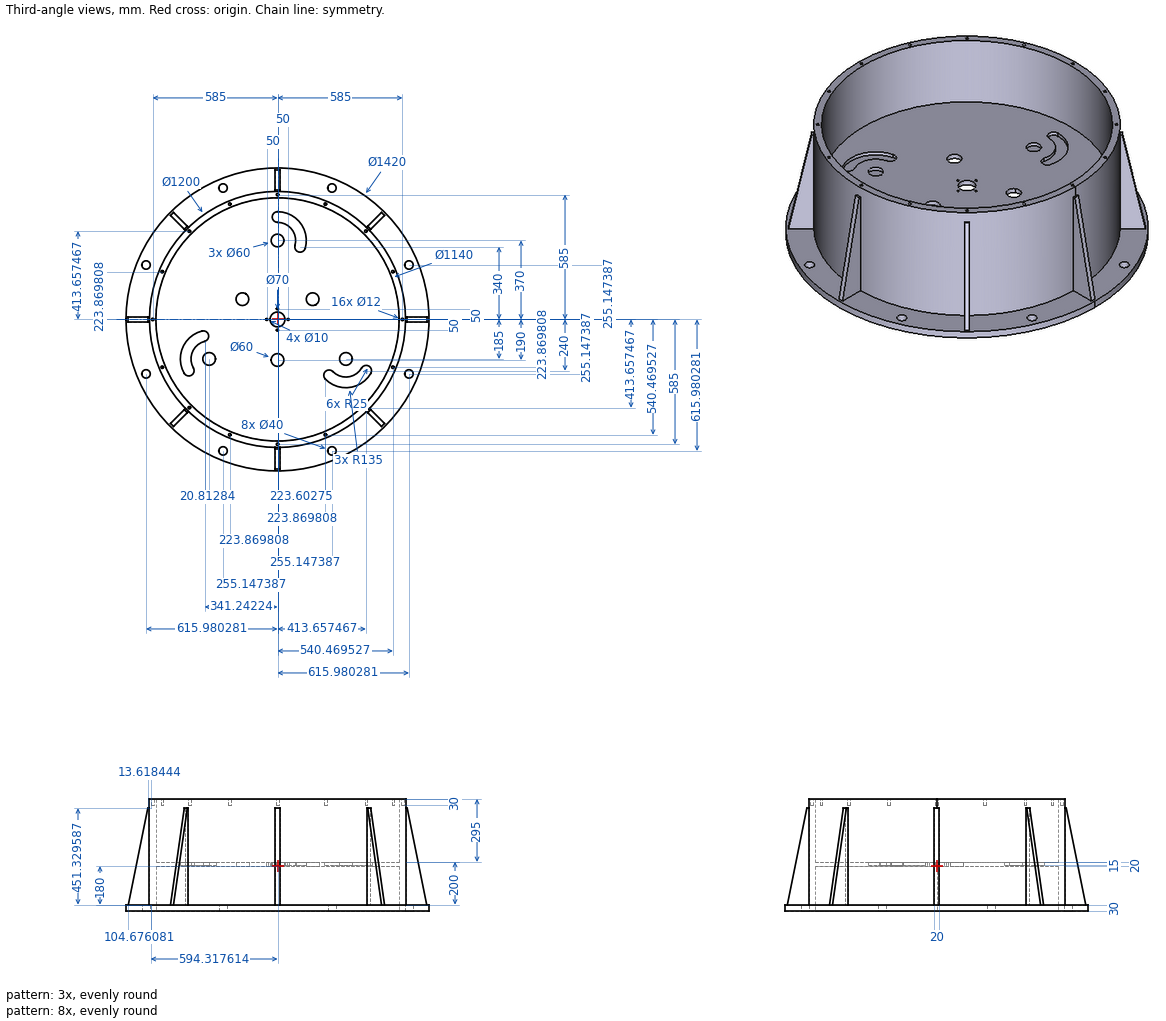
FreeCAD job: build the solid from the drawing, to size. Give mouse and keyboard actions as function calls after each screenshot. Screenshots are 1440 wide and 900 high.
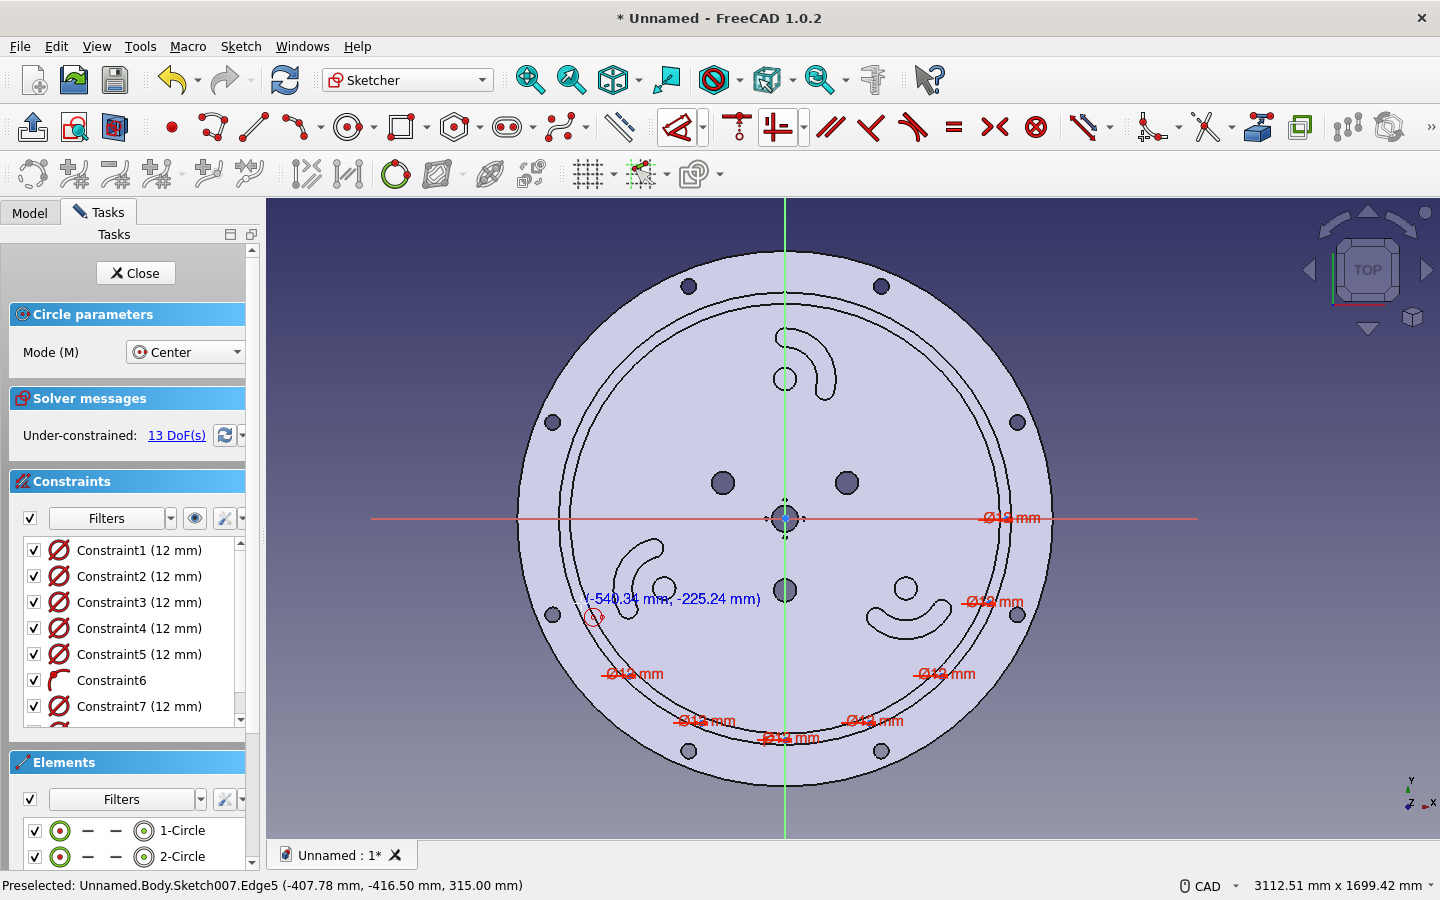
click(581, 603)
move(583, 602)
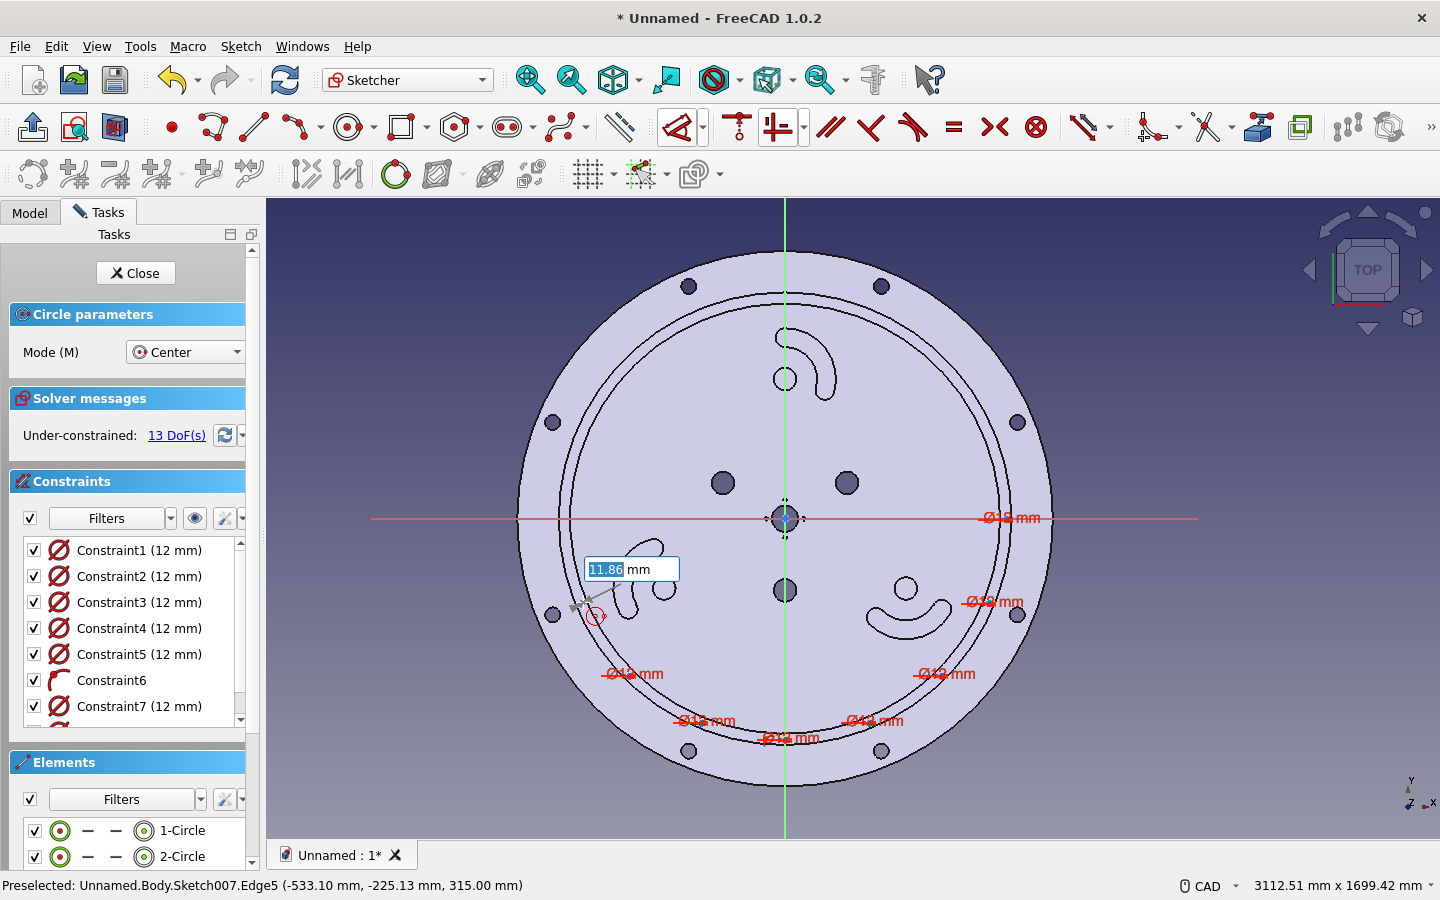
text(12)
key(Return)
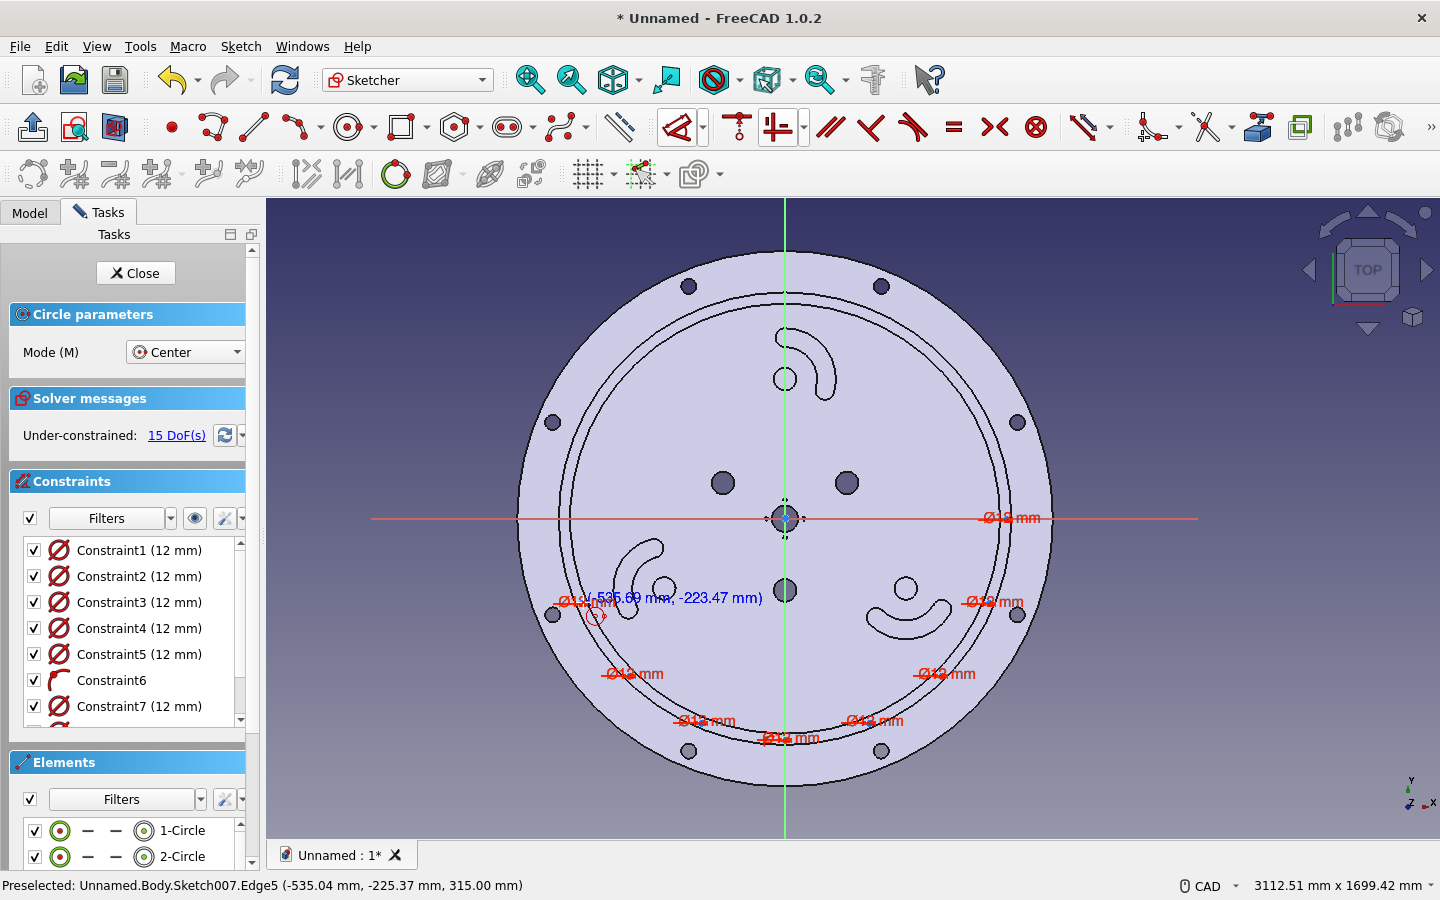
scroll(564, 519, up, 12)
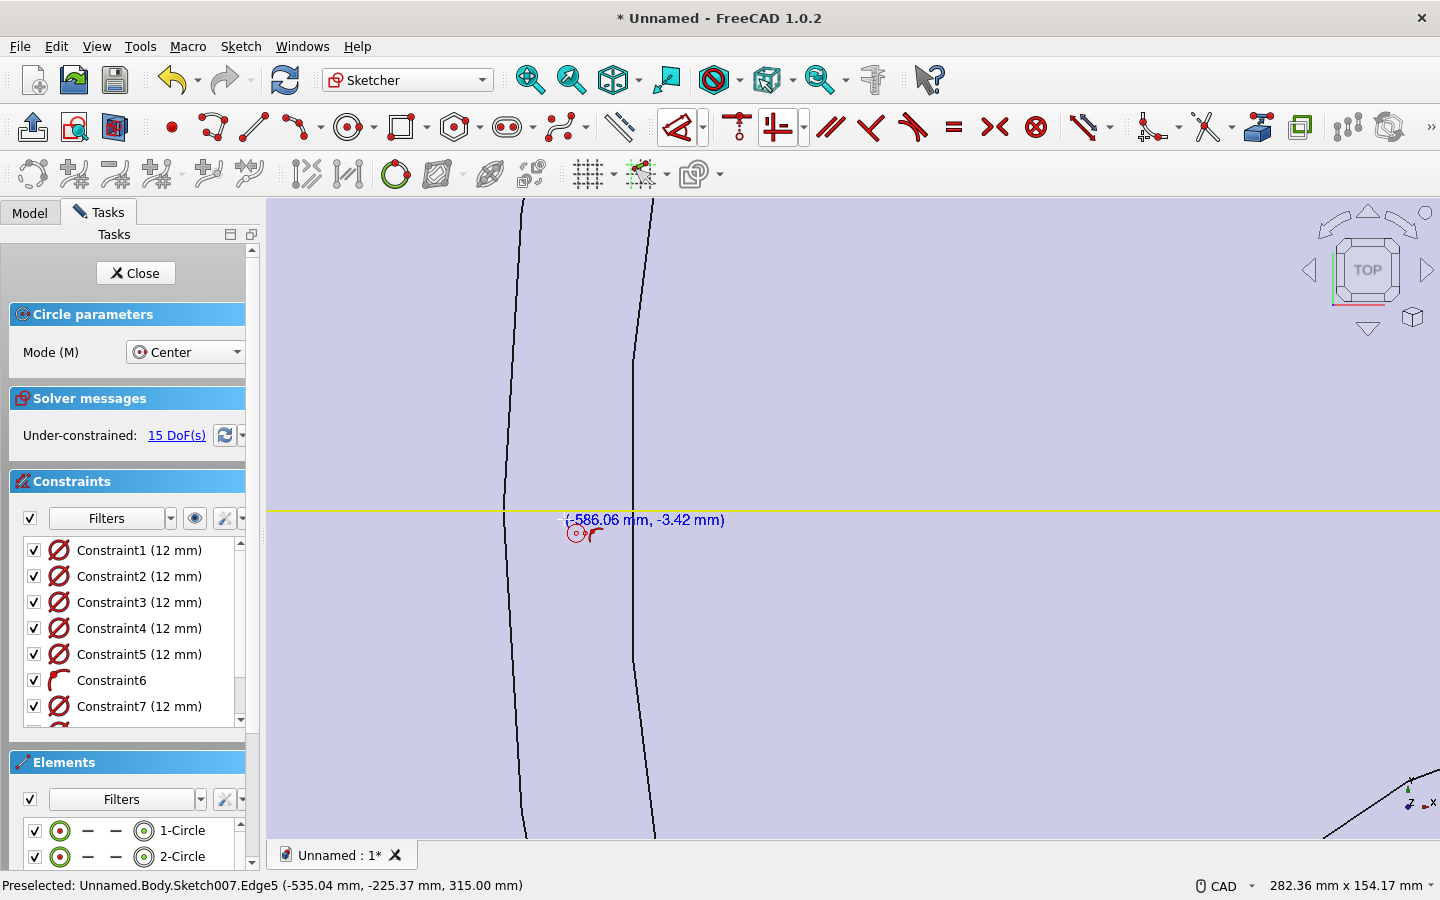
scroll(564, 519, down, 12)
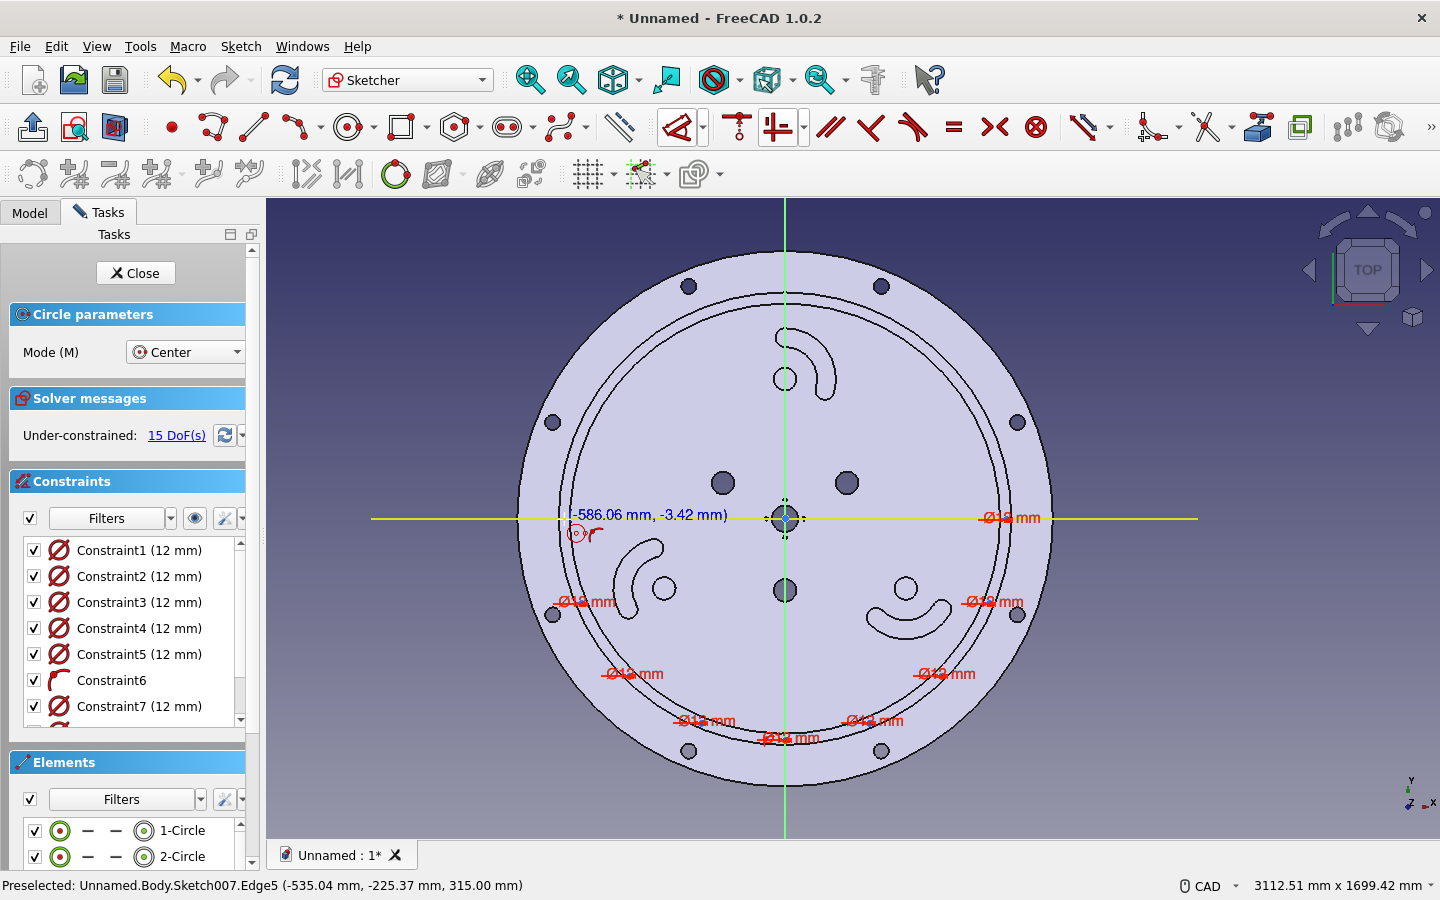
click(564, 519)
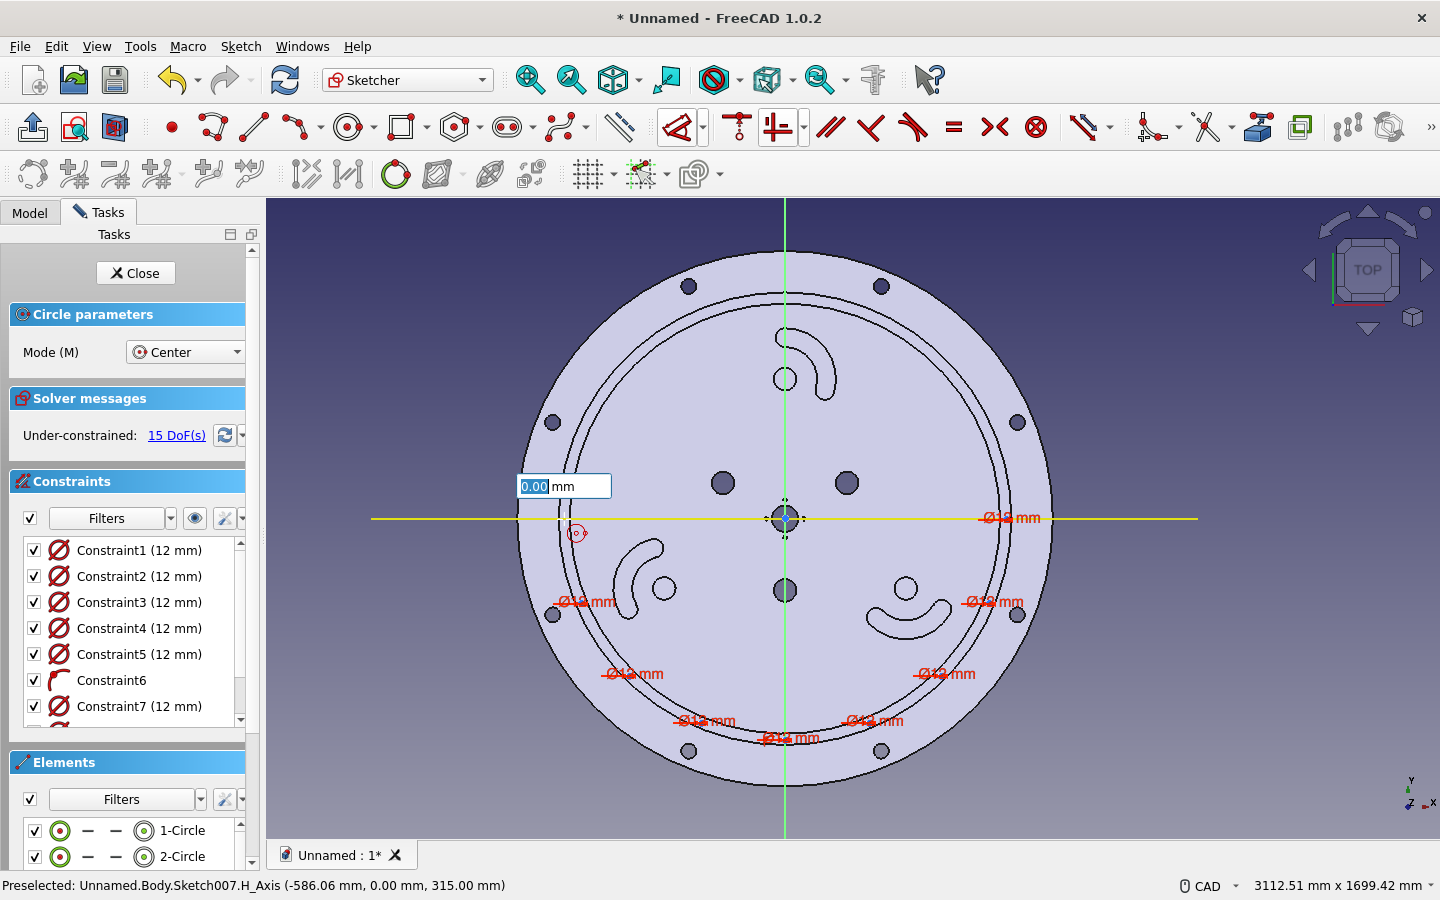
scroll(564, 521, up, 11)
move(559, 515)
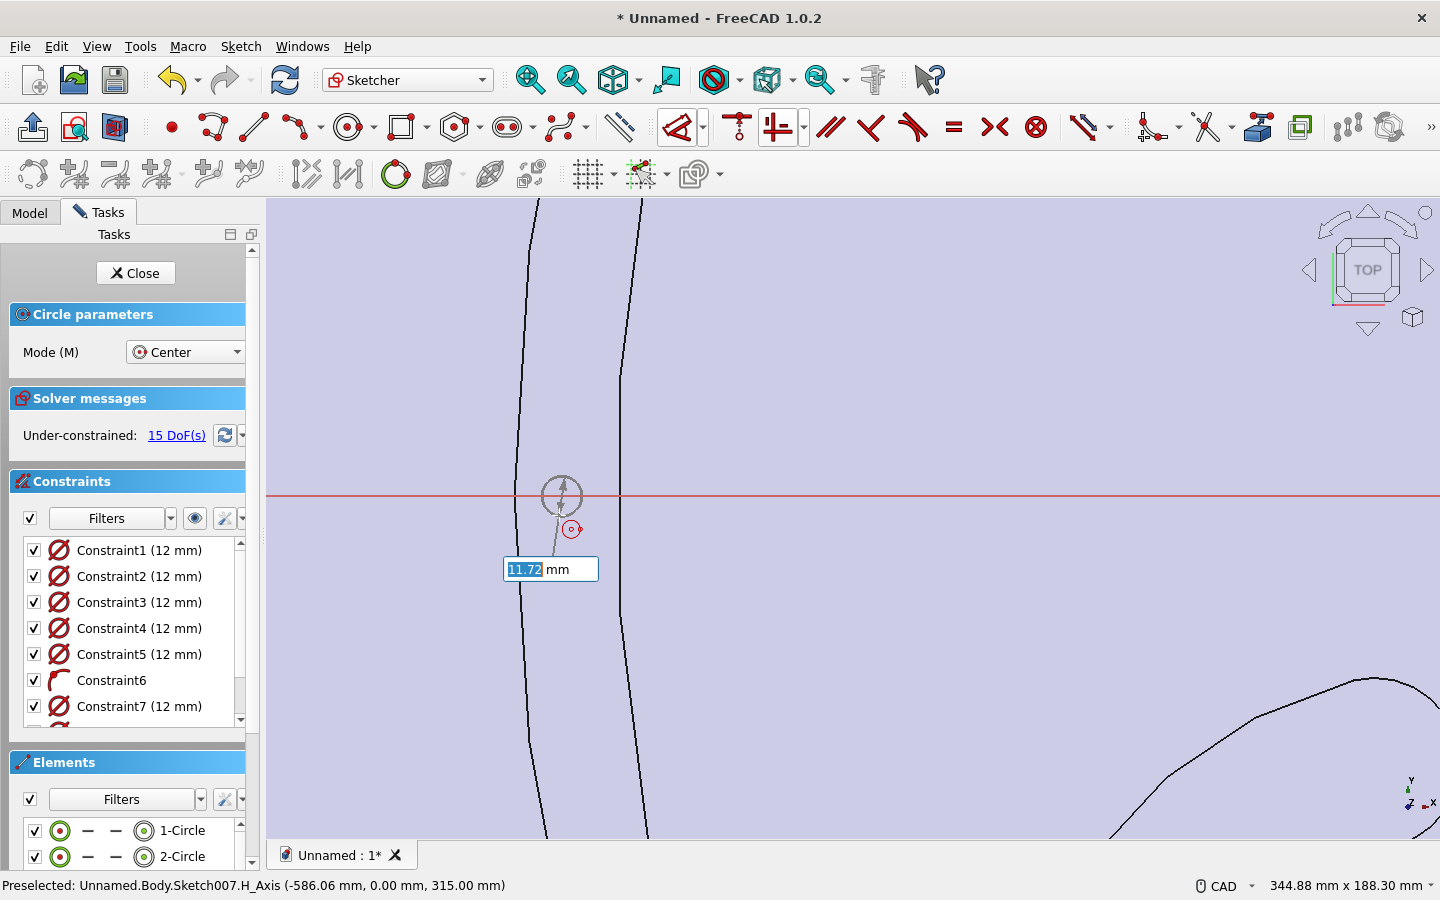
text(12)
key(Return)